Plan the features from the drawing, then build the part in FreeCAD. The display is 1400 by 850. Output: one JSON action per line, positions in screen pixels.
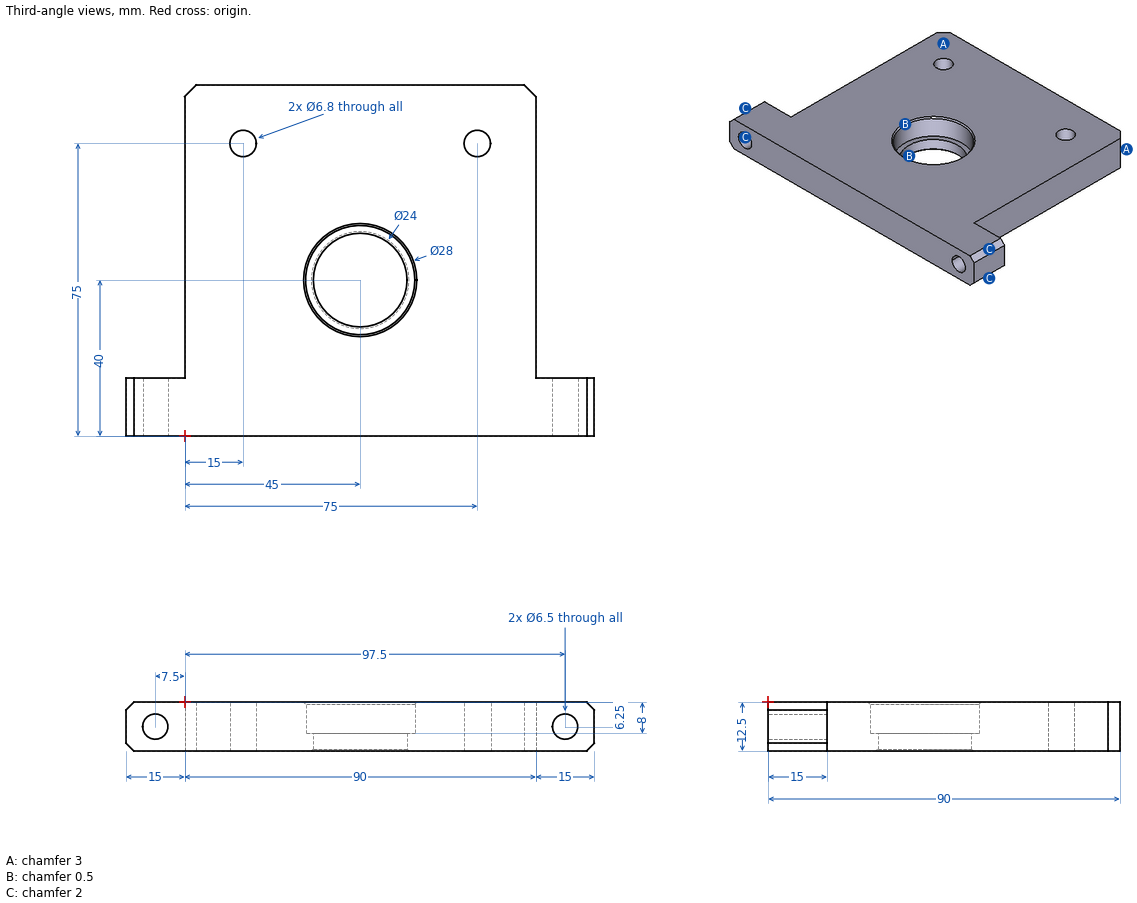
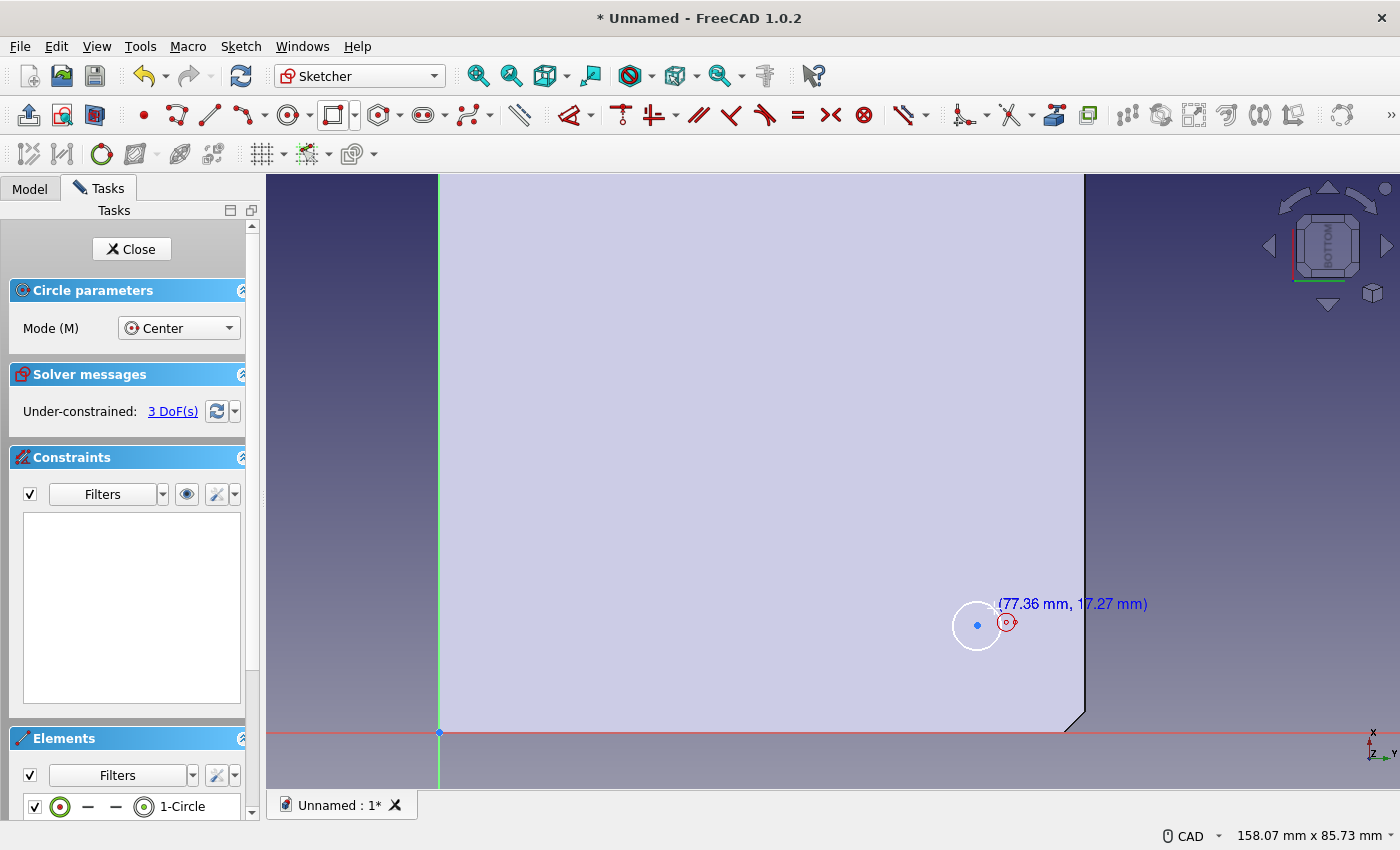
{"action": "scroll", "coordinate": [854, 542], "scroll_direction": "down", "scroll_amount": 2}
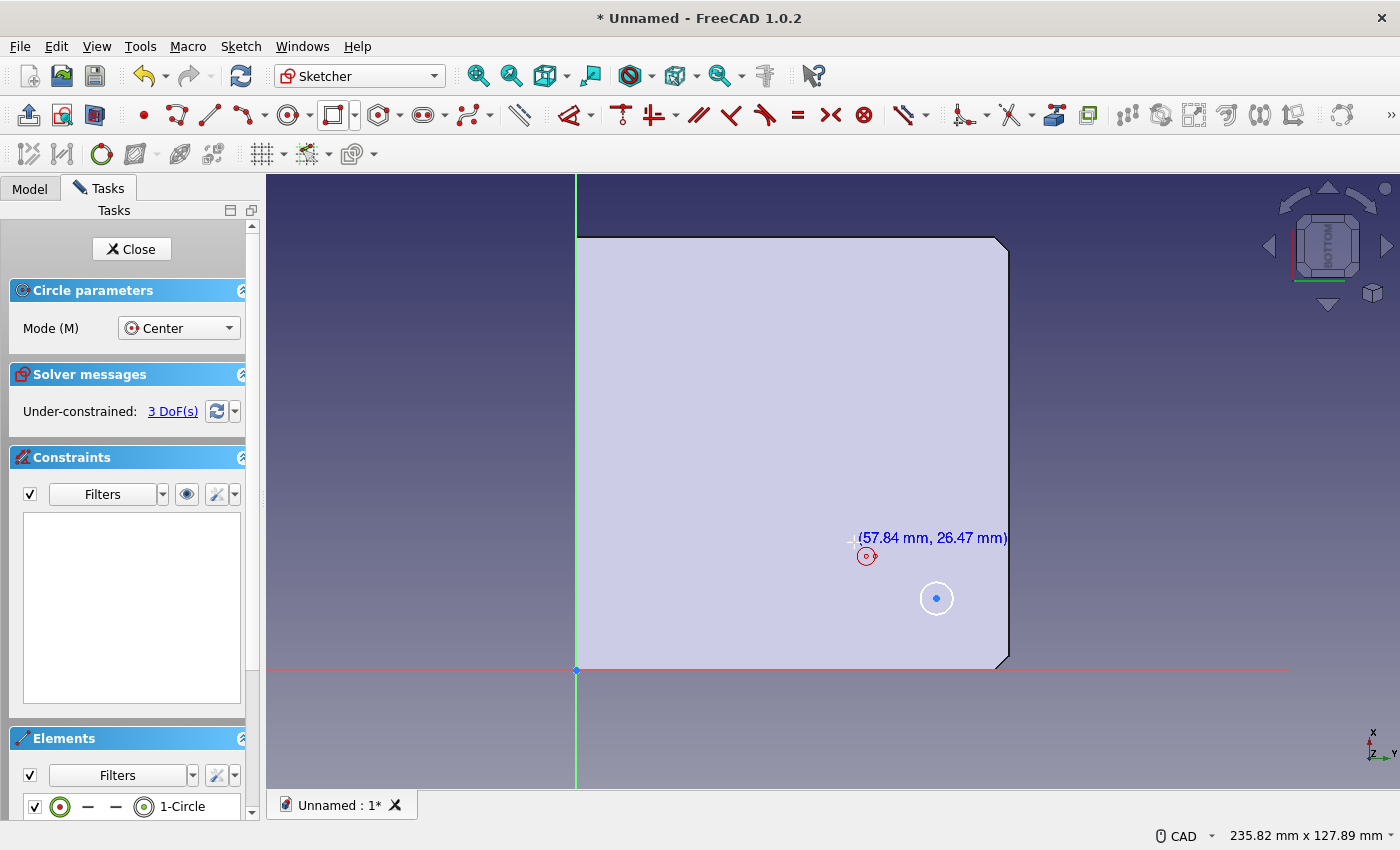
{"action": "scroll", "coordinate": [937, 309], "scroll_direction": "up", "scroll_amount": 2}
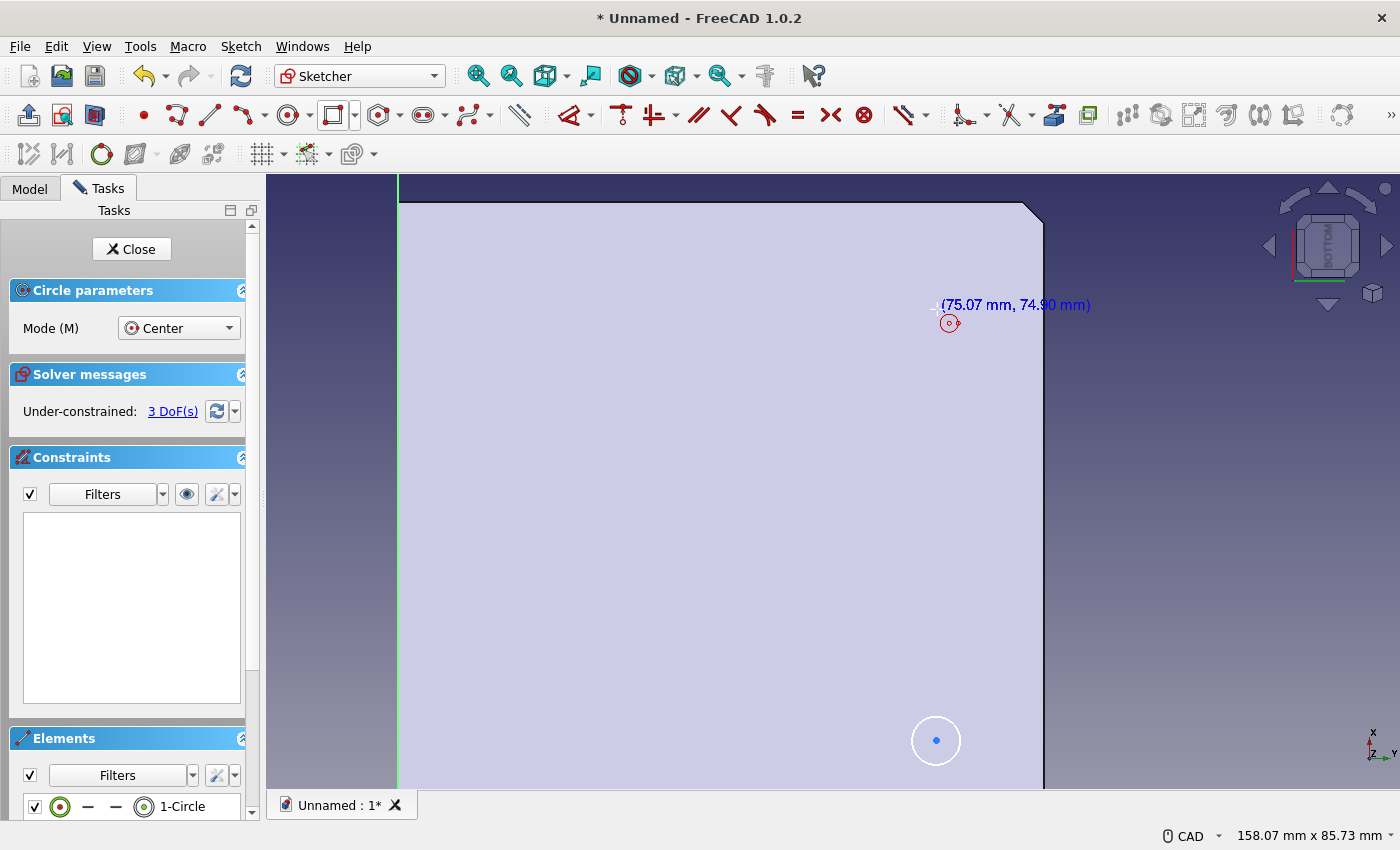
{"action": "left_click", "coordinate": [936, 310]}
{"action": "left_click", "coordinate": [953, 292]}
{"action": "key", "text": "Escape"}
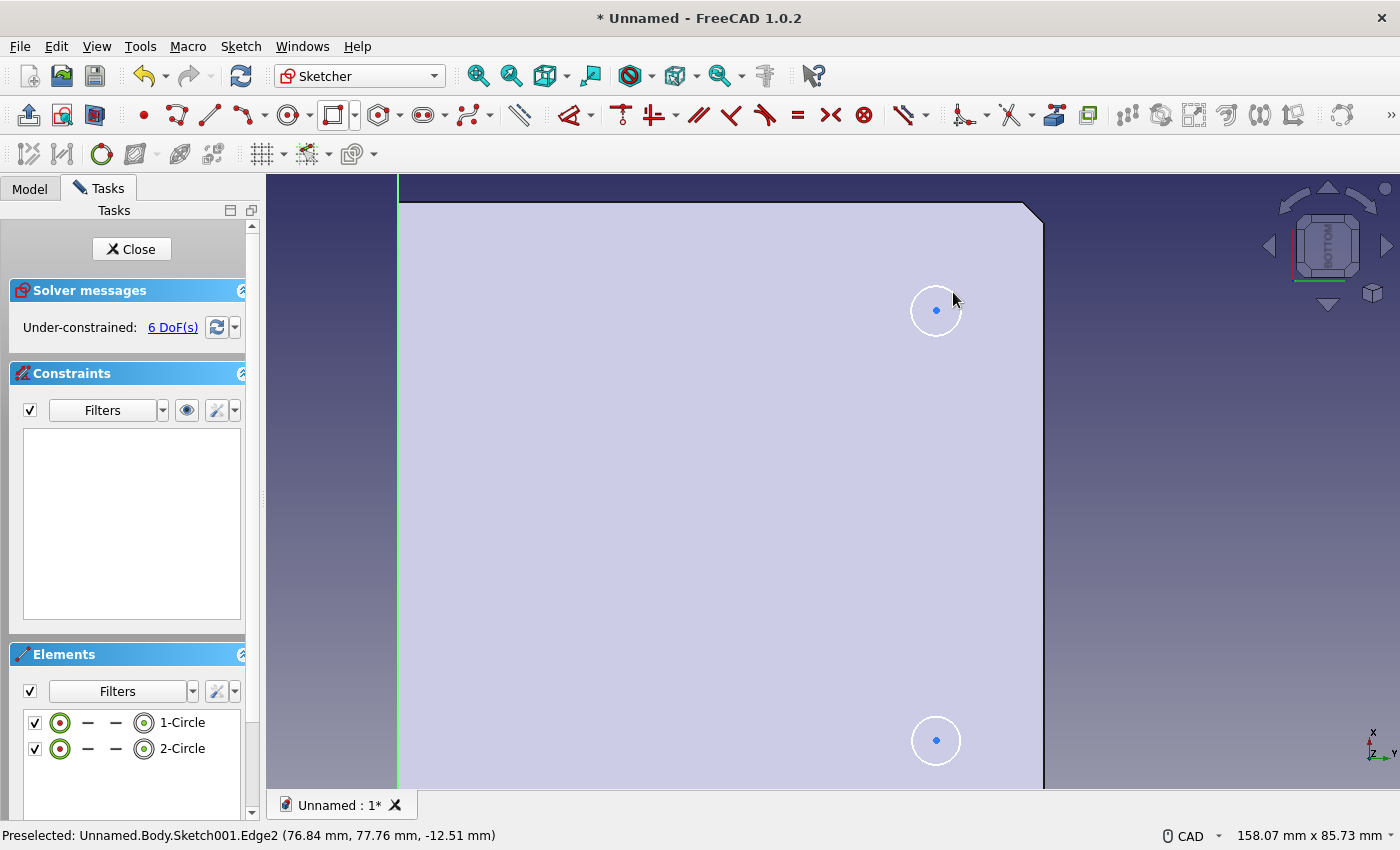
{"action": "left_click", "coordinate": [953, 724]}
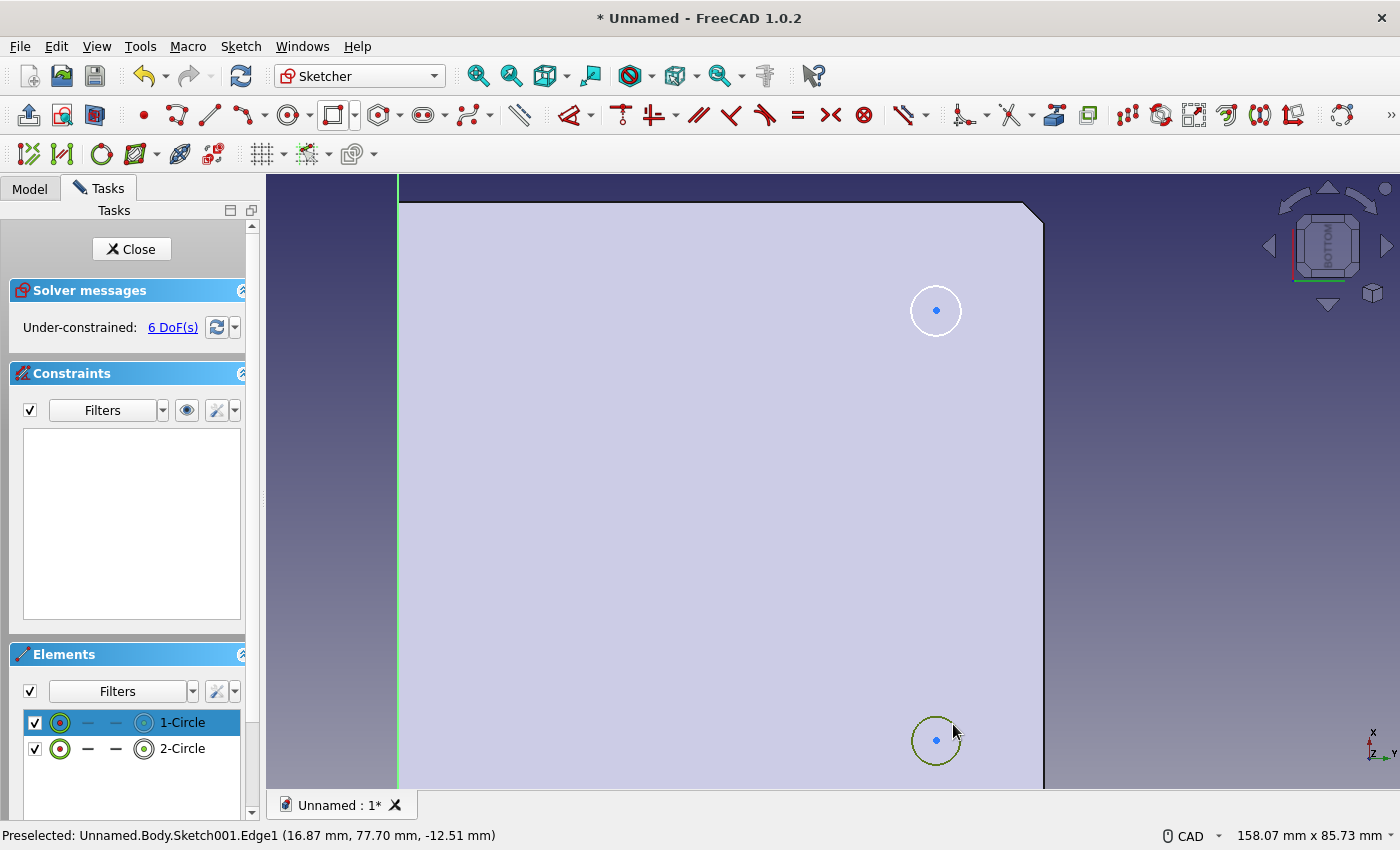
{"action": "left_click", "coordinate": [953, 293]}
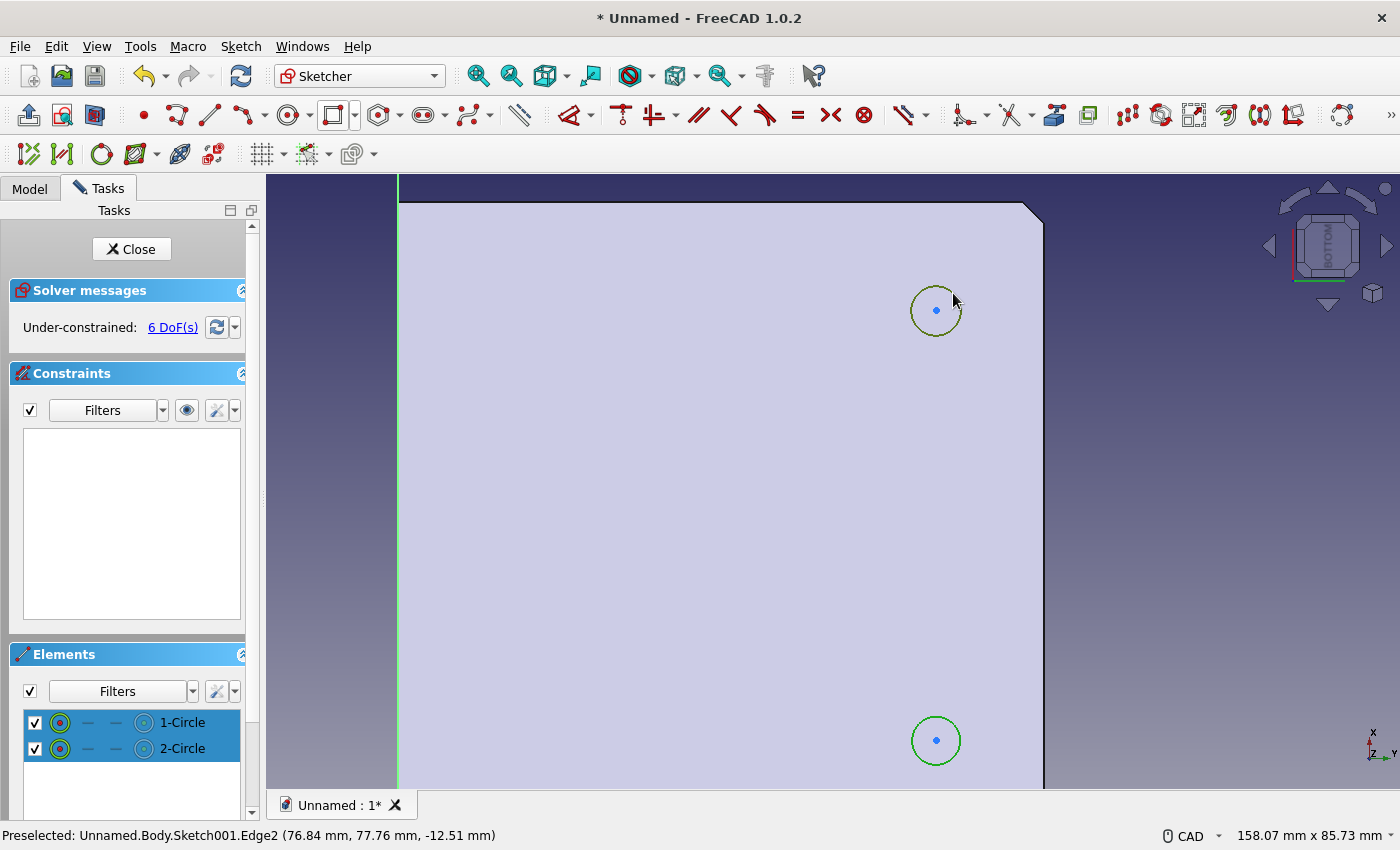
{"action": "left_click", "coordinate": [798, 116]}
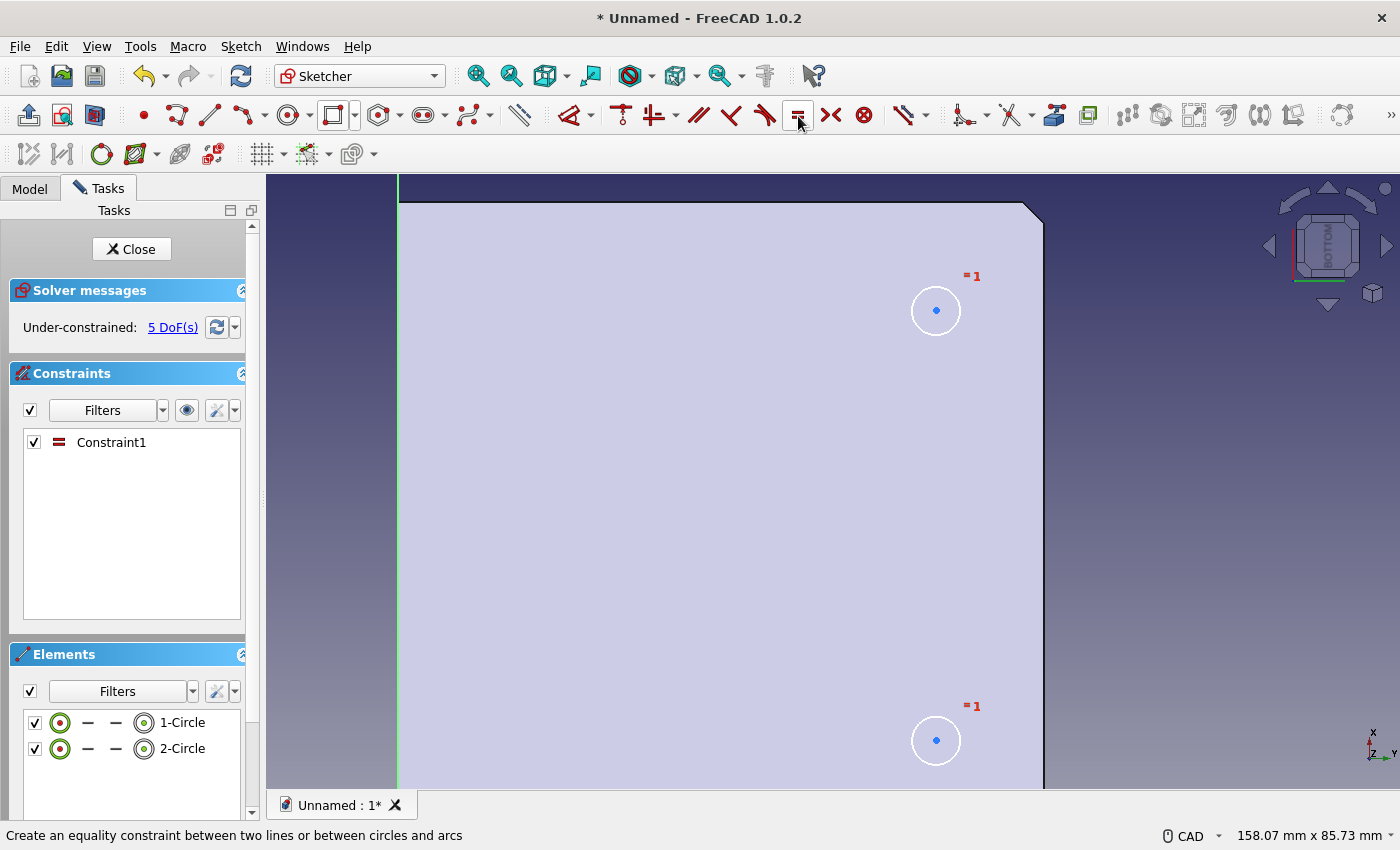
{"action": "left_click", "coordinate": [568, 116]}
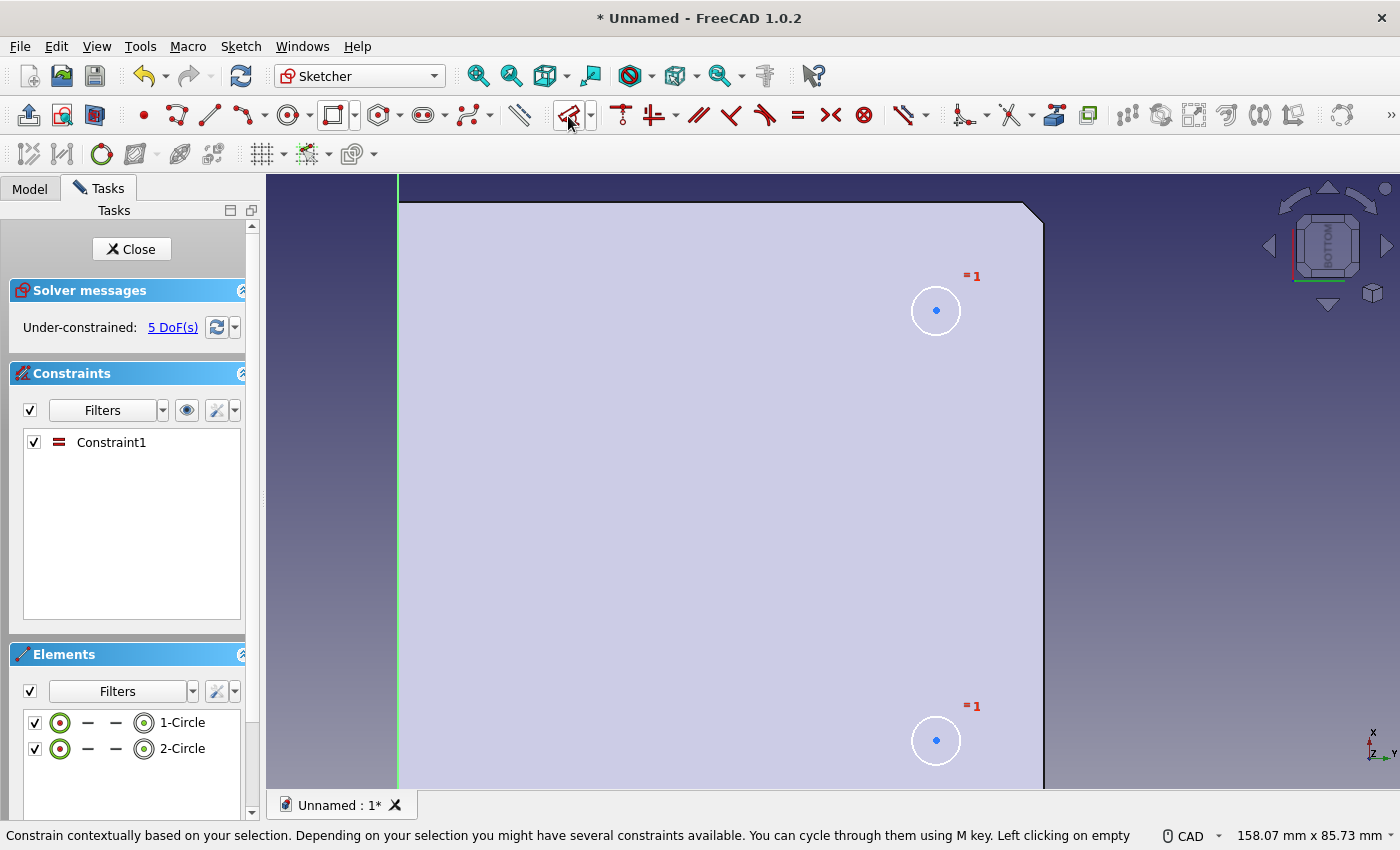
{"action": "left_click", "coordinate": [953, 724]}
{"action": "left_click", "coordinate": [976, 701]}